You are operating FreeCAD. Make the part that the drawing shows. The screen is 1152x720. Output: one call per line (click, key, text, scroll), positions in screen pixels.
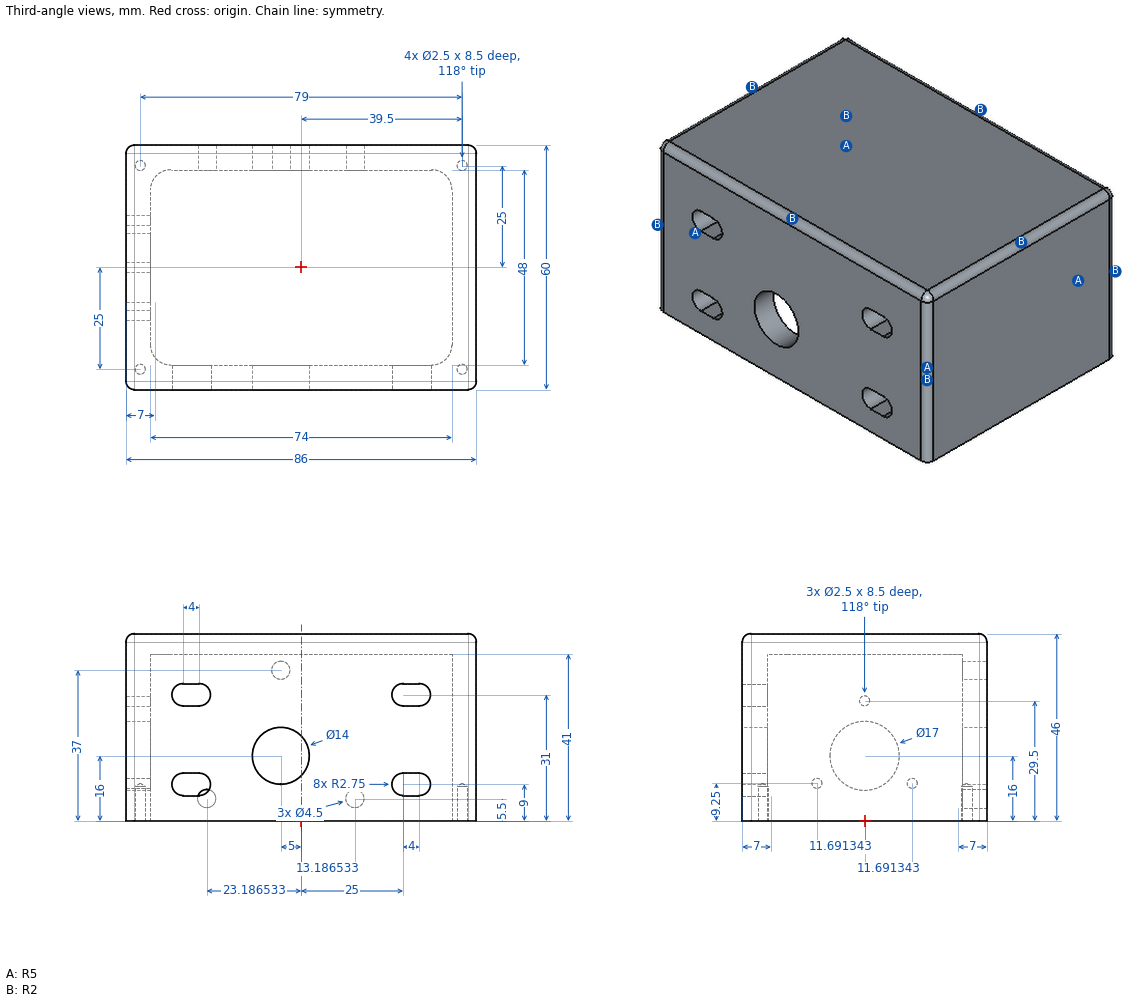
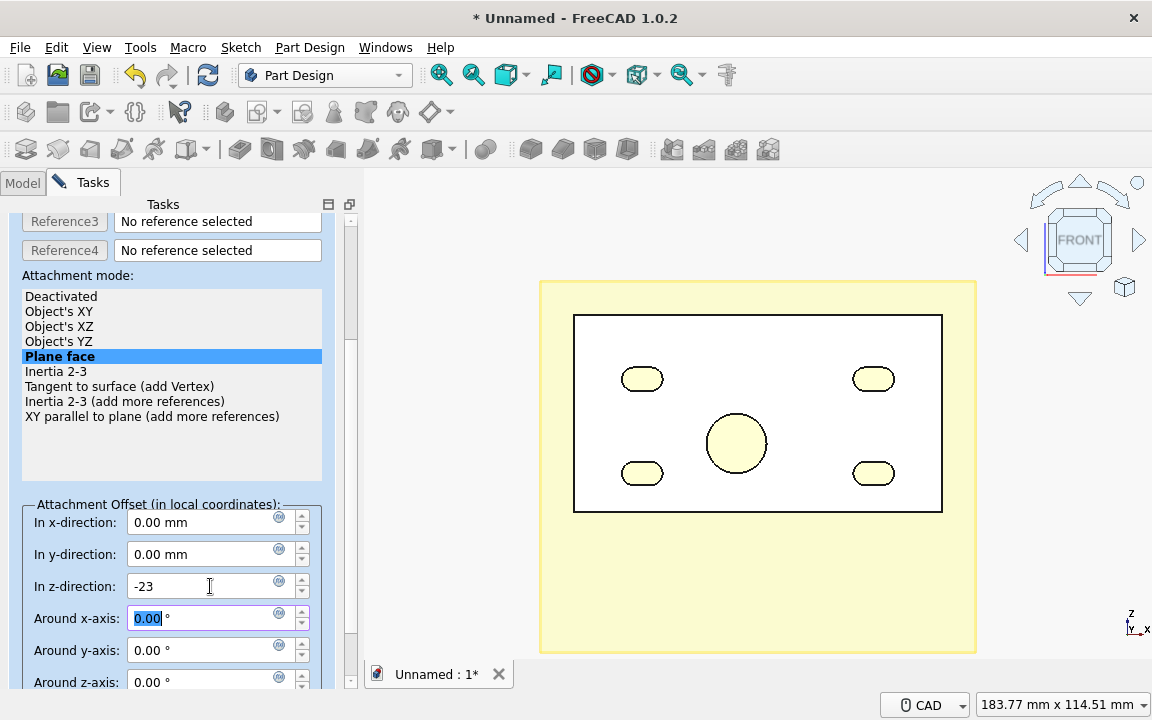
scroll(351, 451, up, 4)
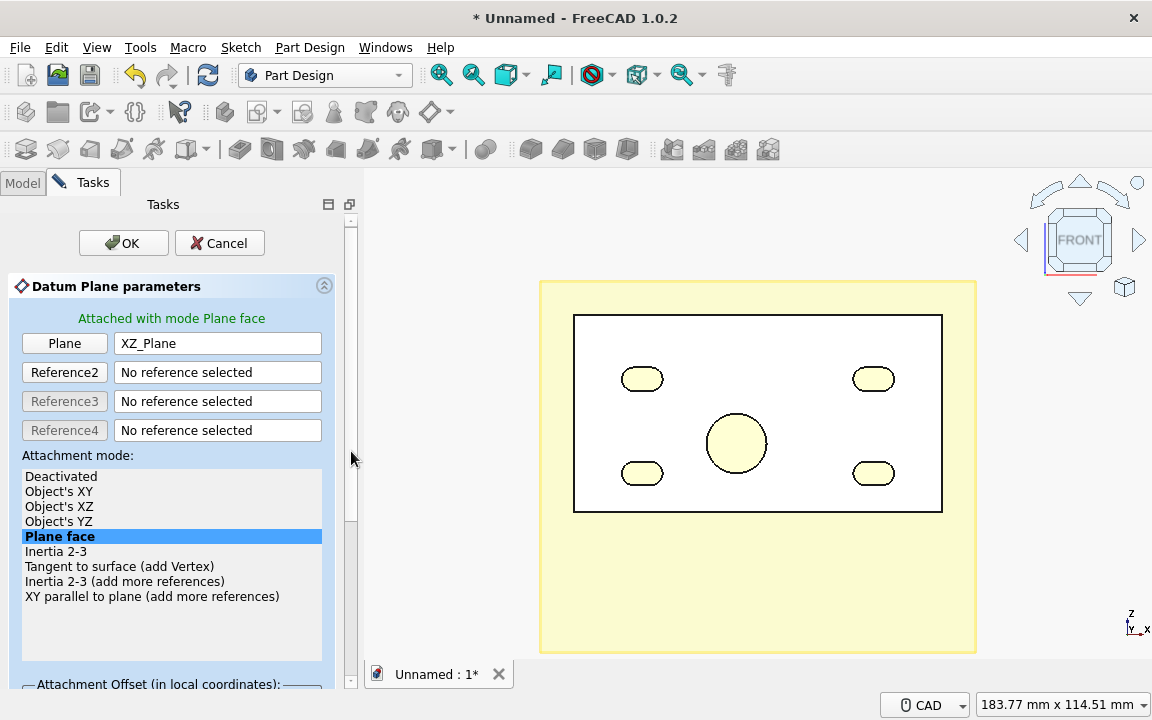
click(124, 243)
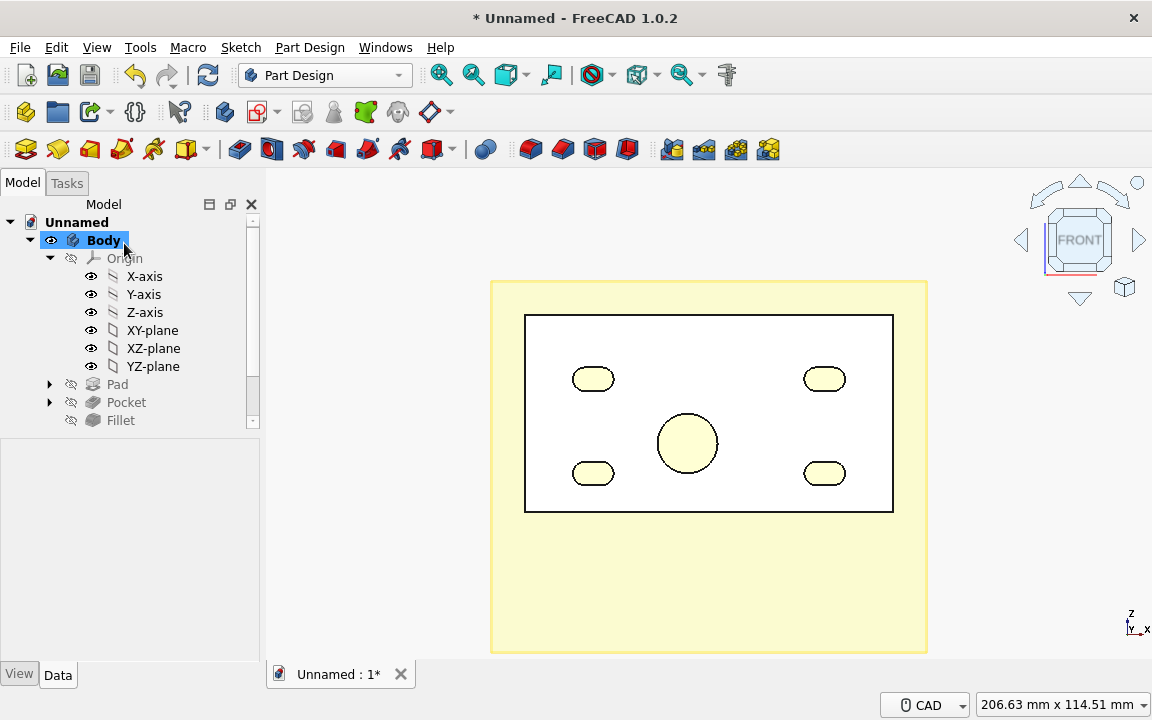
scroll(100, 326, down, 3)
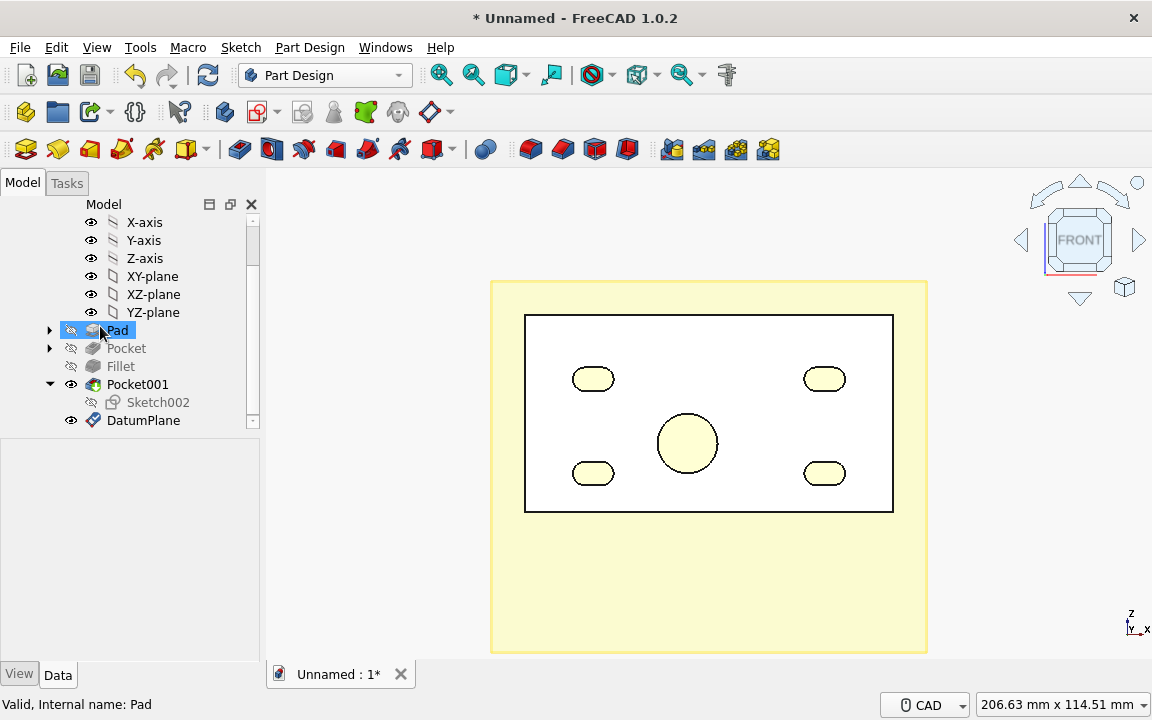
click(116, 420)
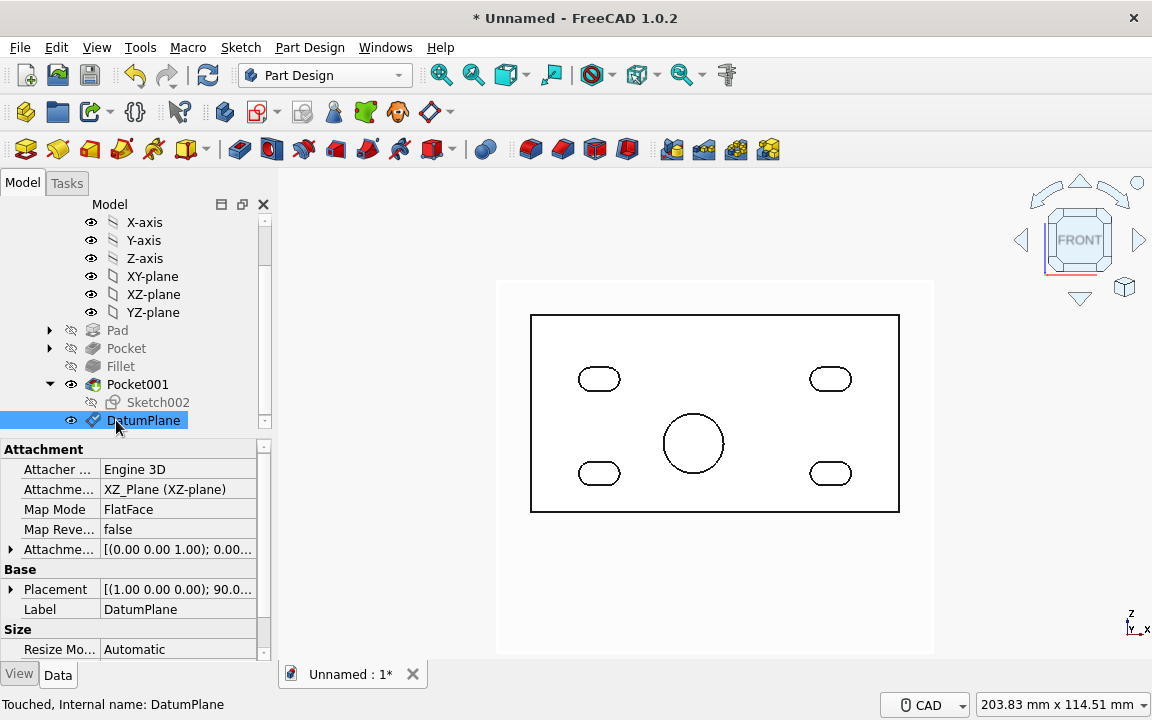
click(258, 112)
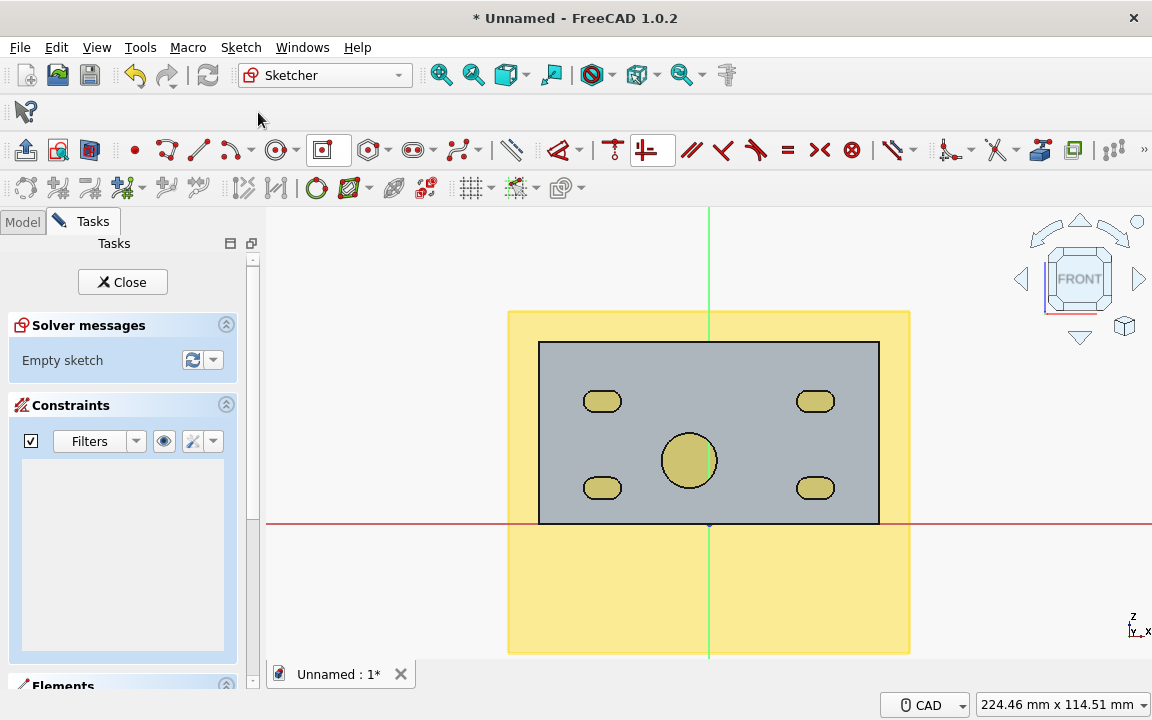
key(q)
key(s)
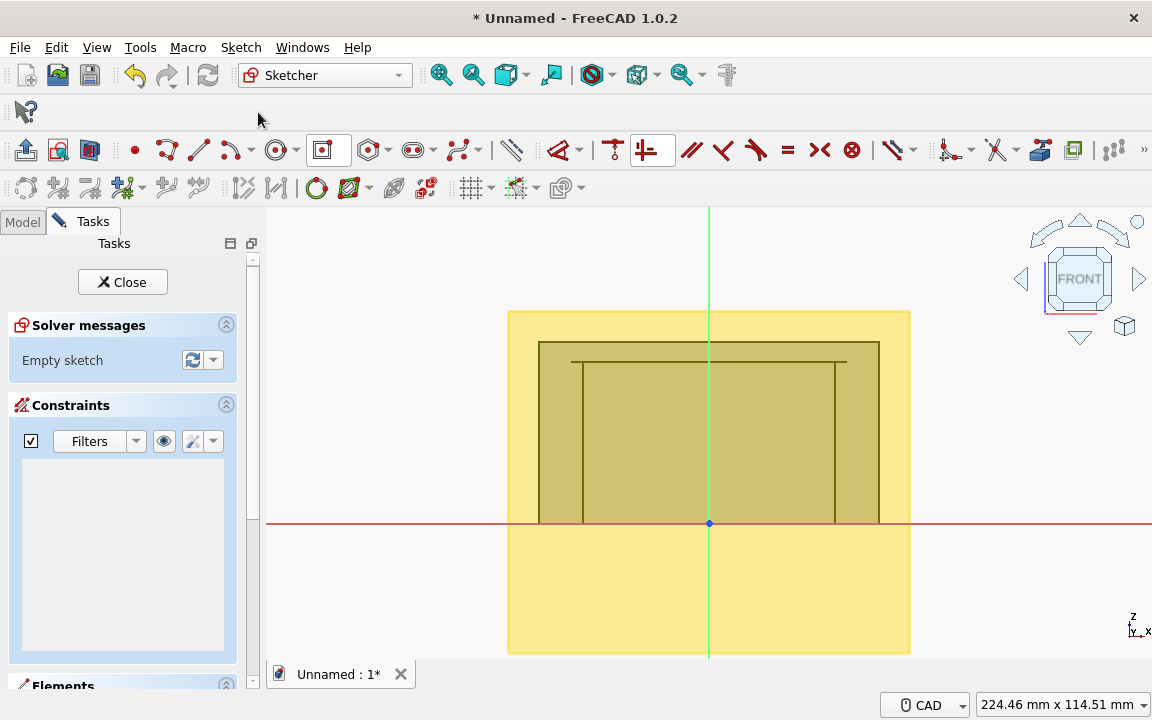
scroll(749, 463, up, 3)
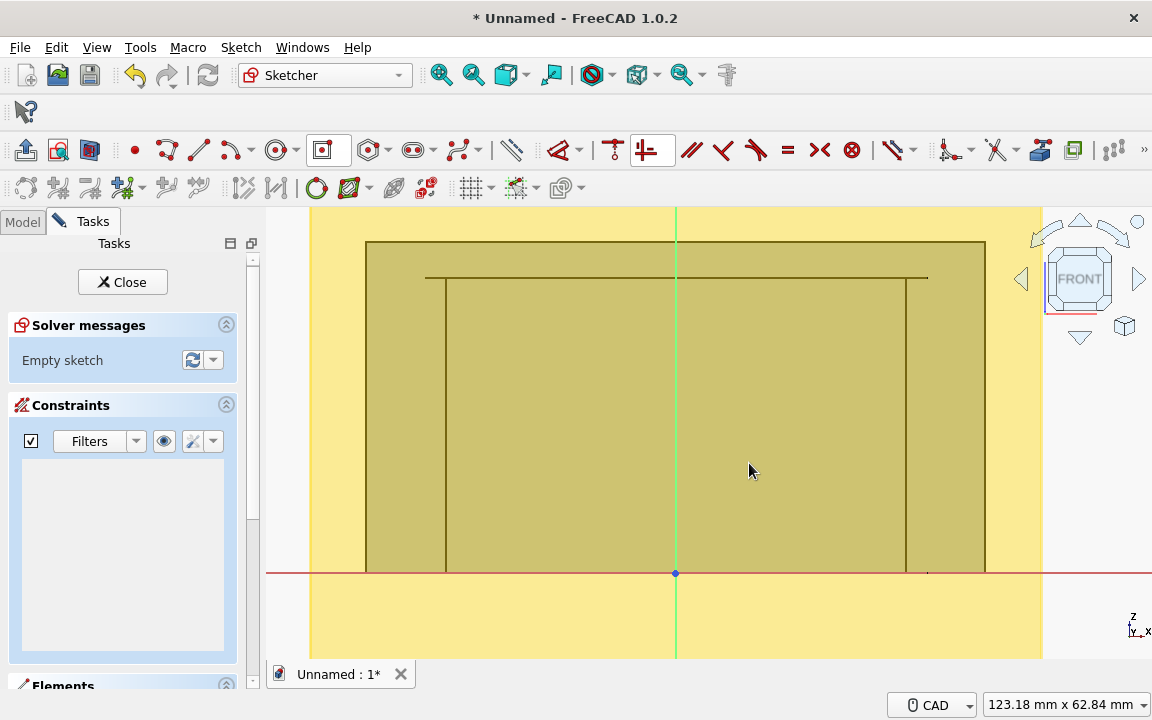
key(g)
key(c)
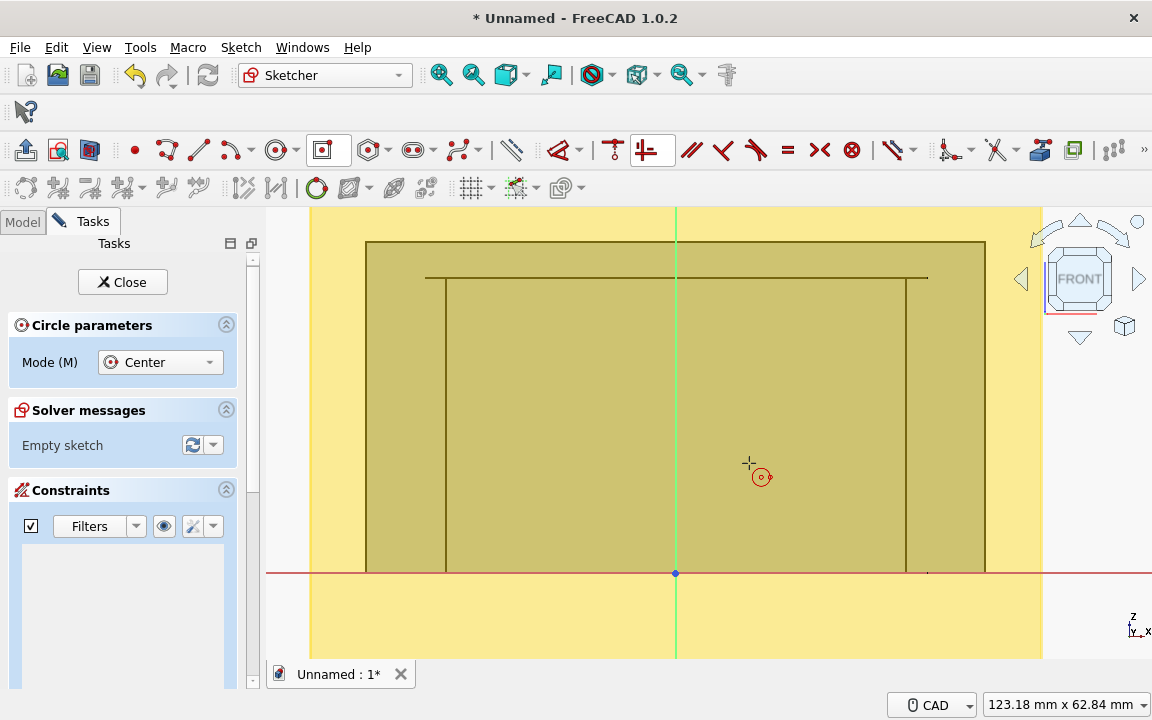
click(640, 458)
click(604, 423)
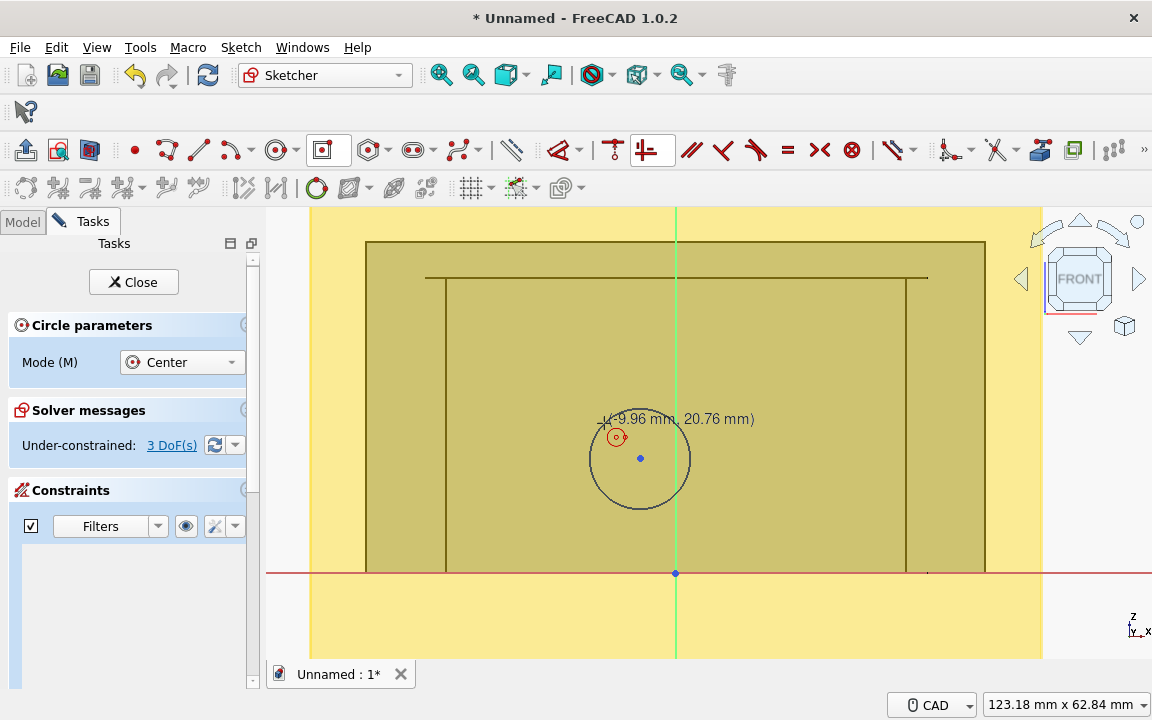
scroll(771, 534, up, 2)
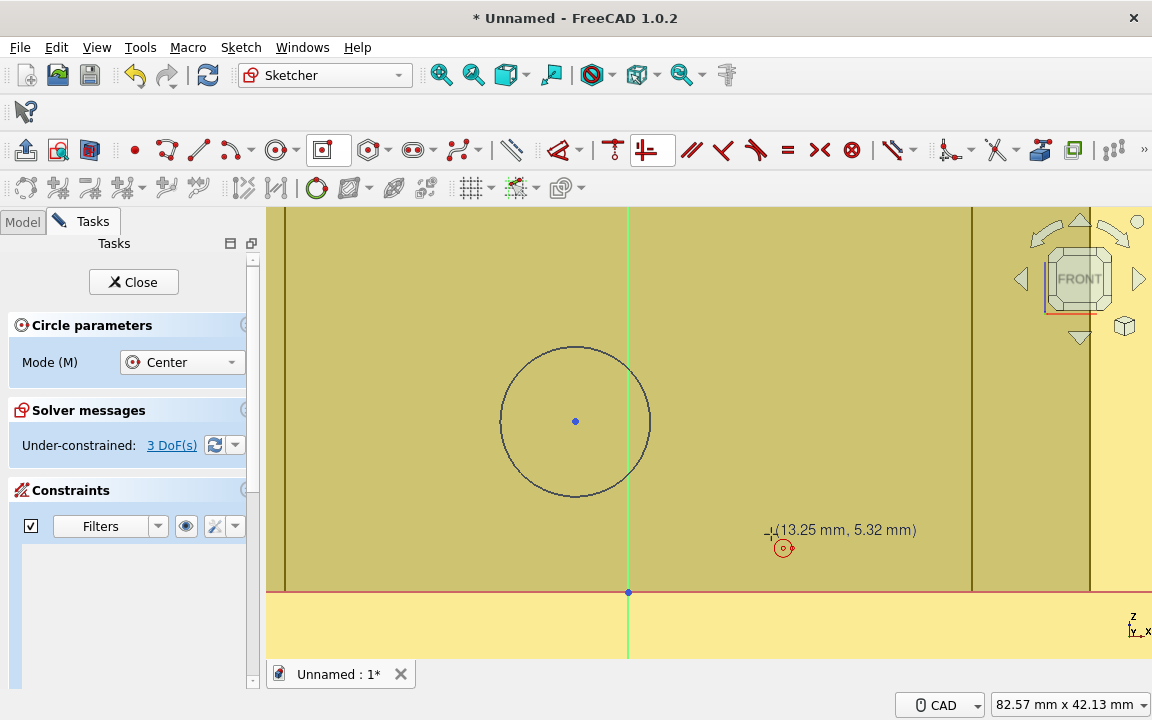
click(770, 533)
click(787, 516)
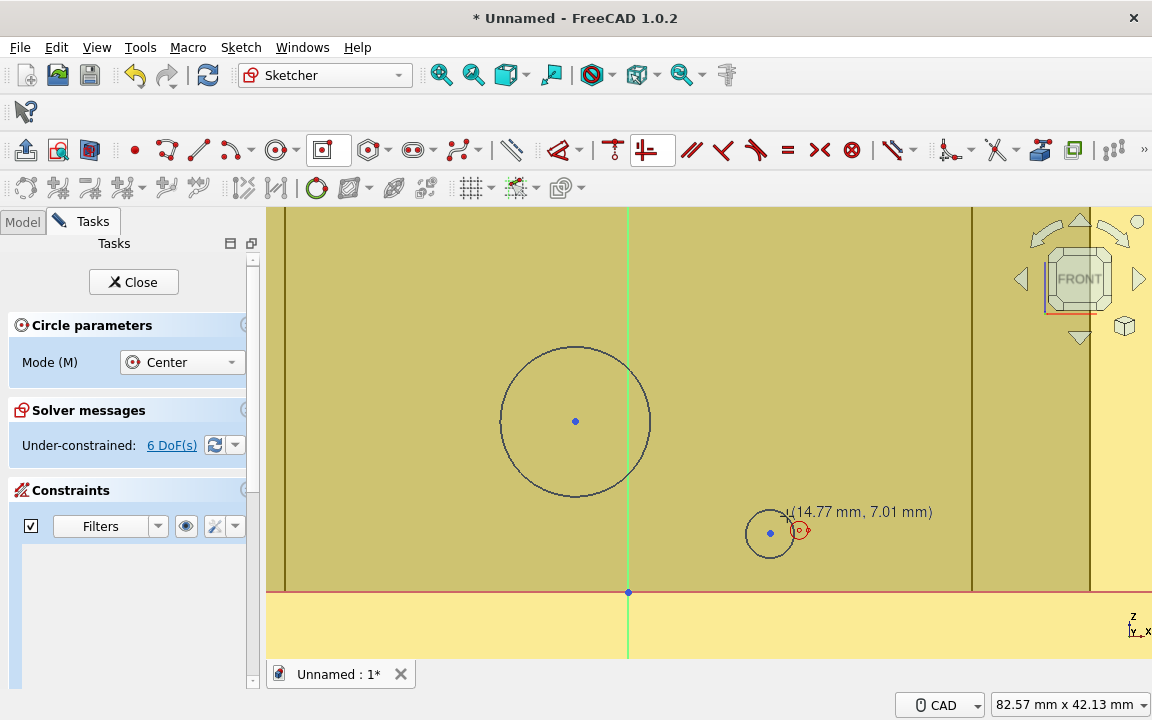
scroll(774, 537, down, 2)